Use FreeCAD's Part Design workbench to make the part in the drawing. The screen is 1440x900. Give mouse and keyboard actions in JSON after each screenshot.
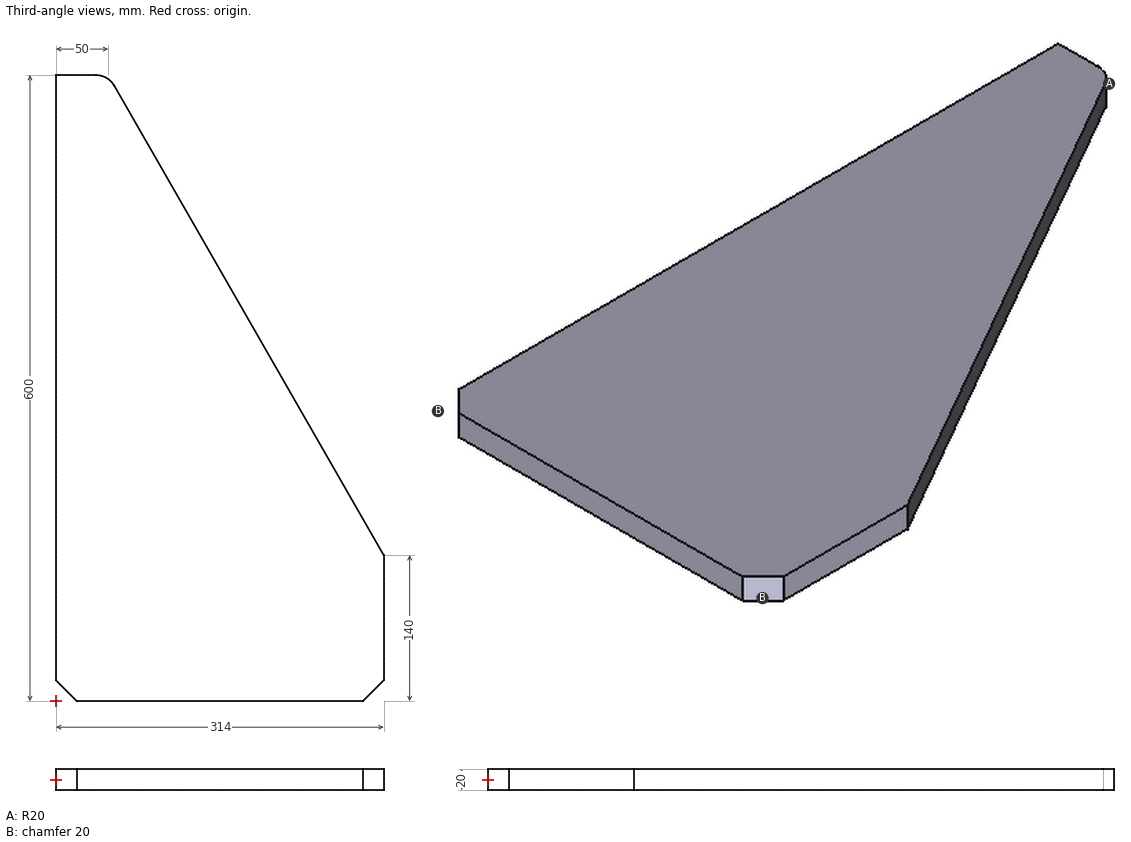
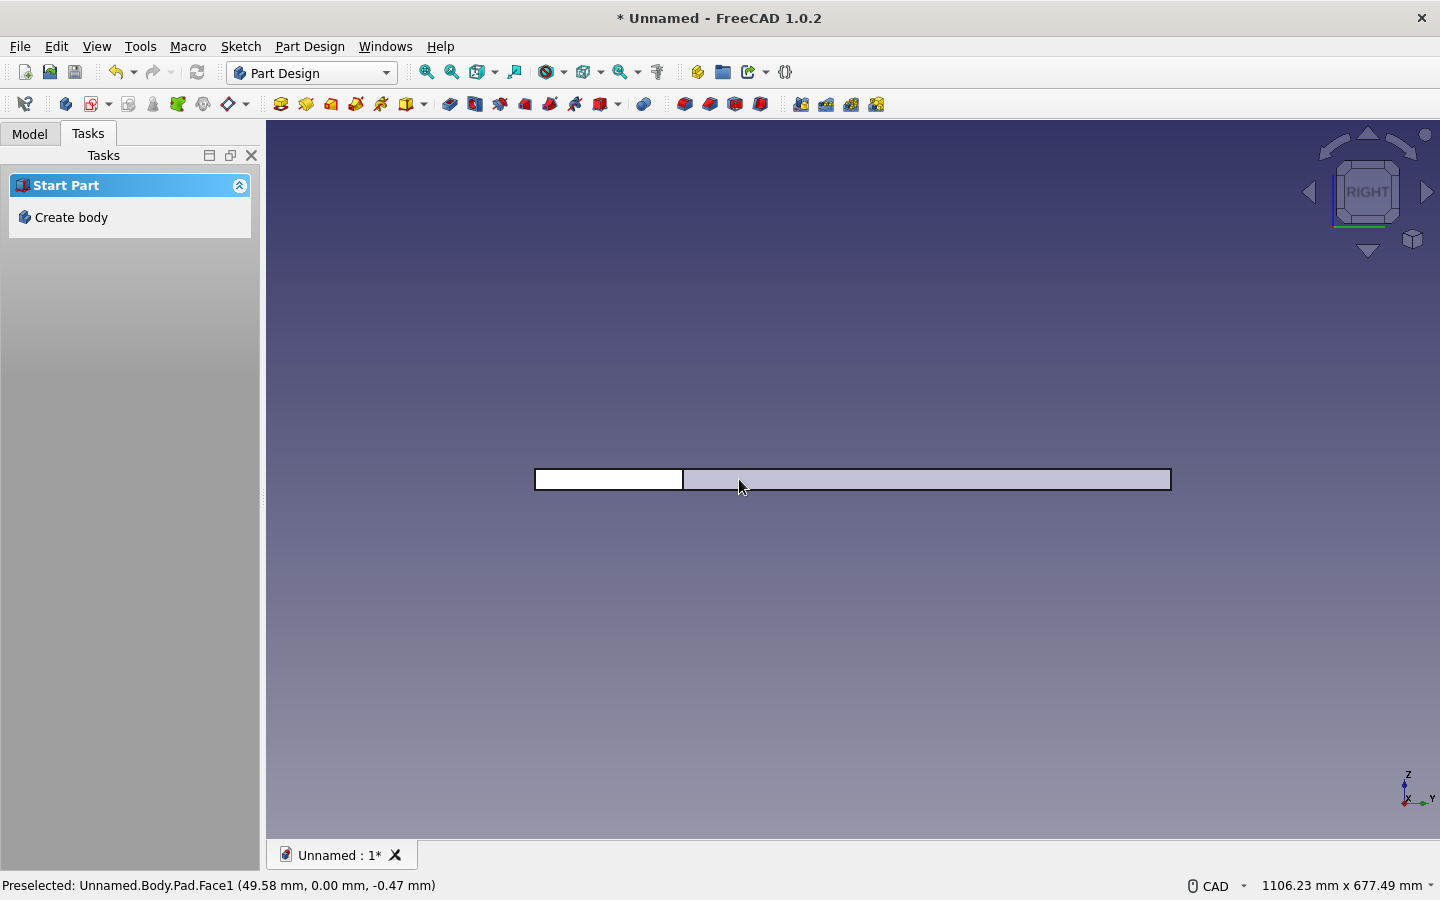
{"action": "scroll", "coordinate": [1171, 478], "scroll_direction": "up", "scroll_amount": 4}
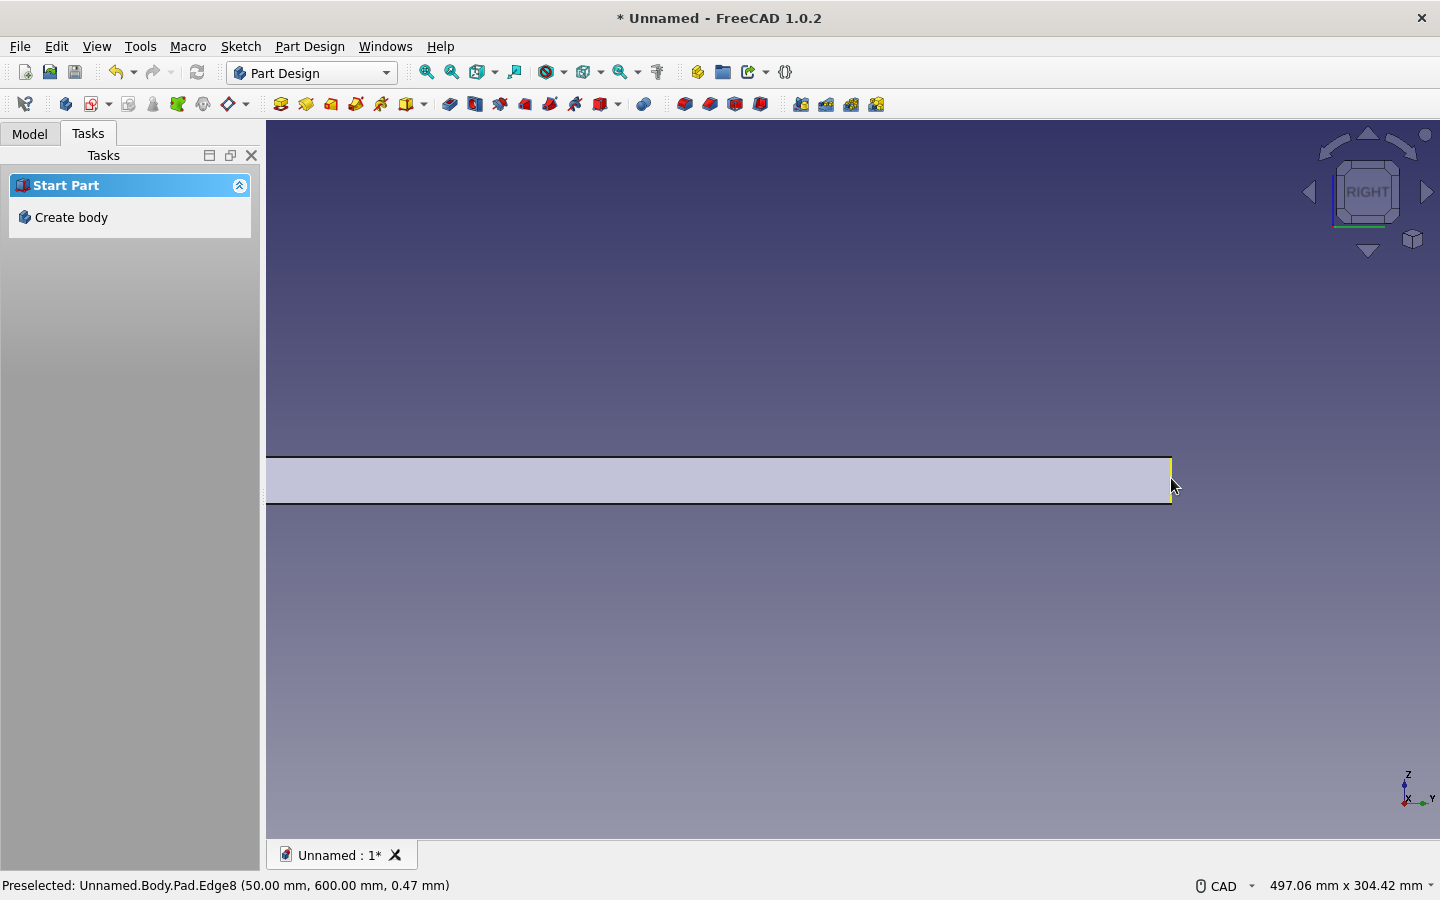
{"action": "key", "text": "v f"}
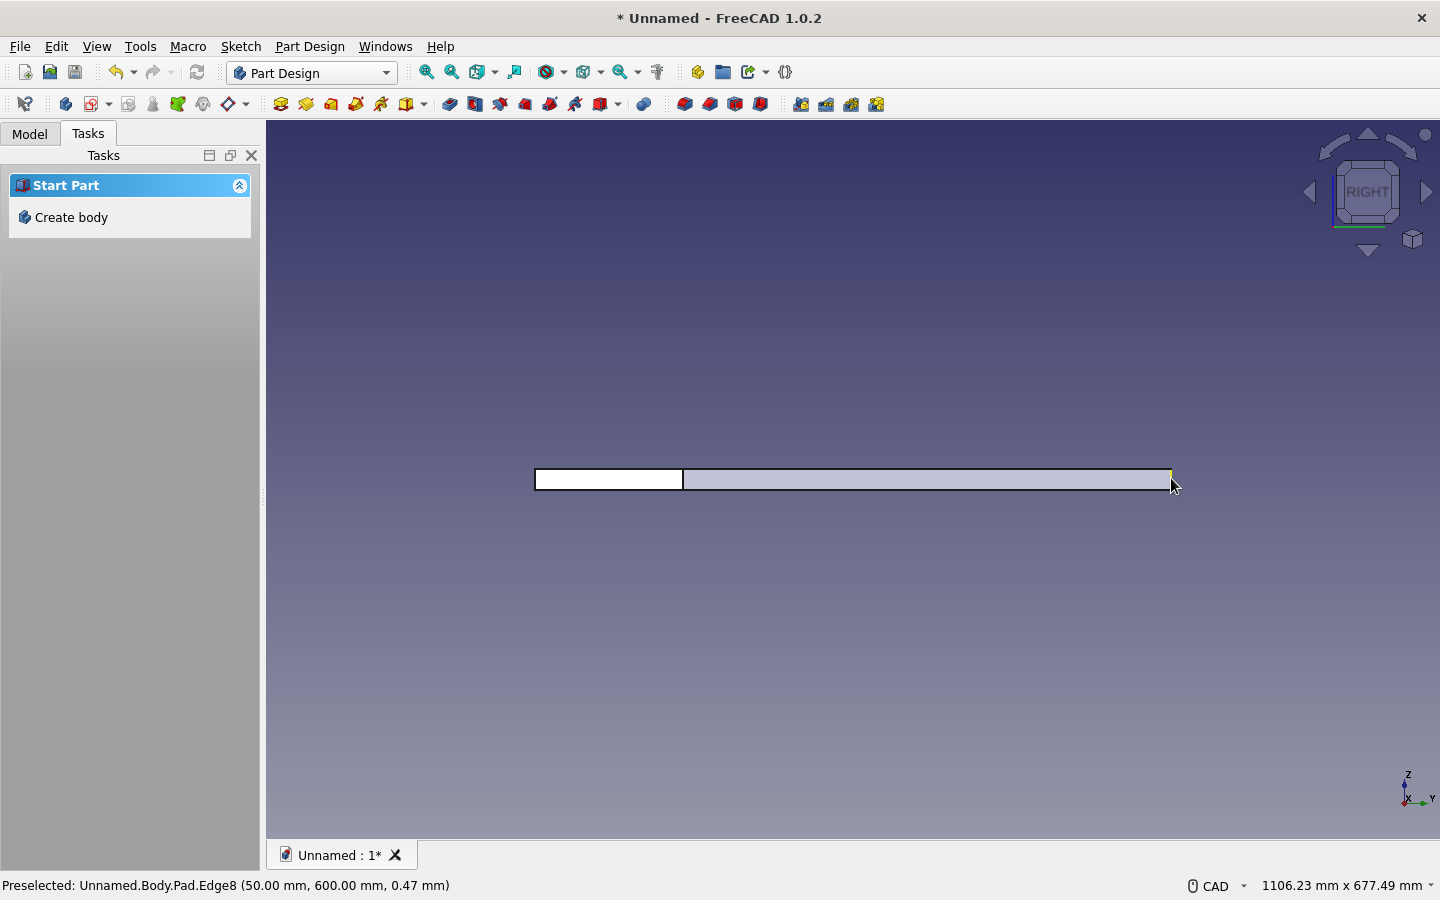
{"action": "key", "text": "5"}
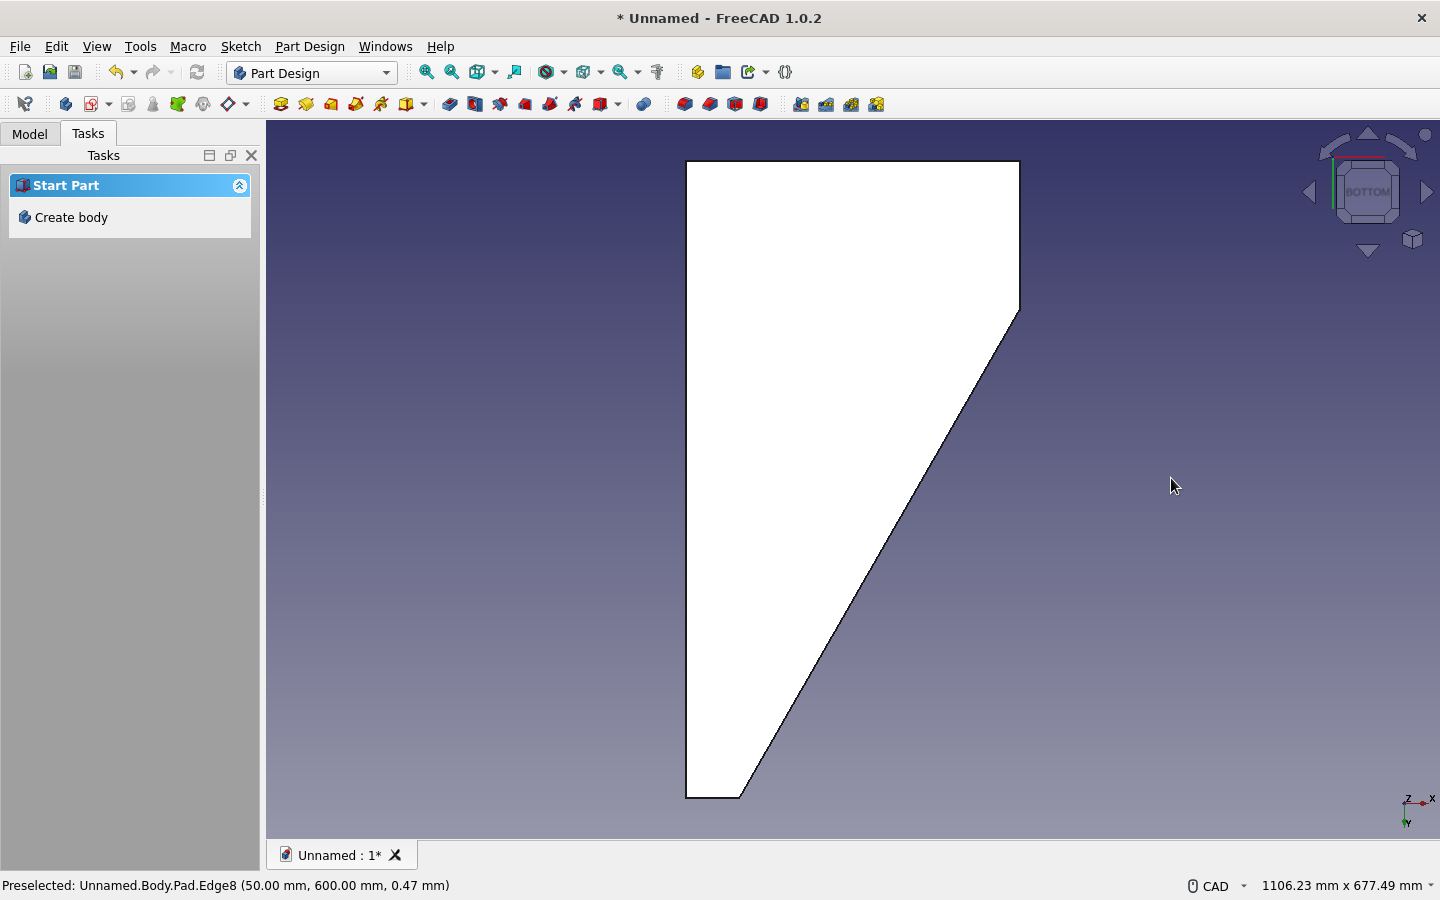
{"action": "scroll", "coordinate": [739, 797], "scroll_direction": "up", "scroll_amount": 4}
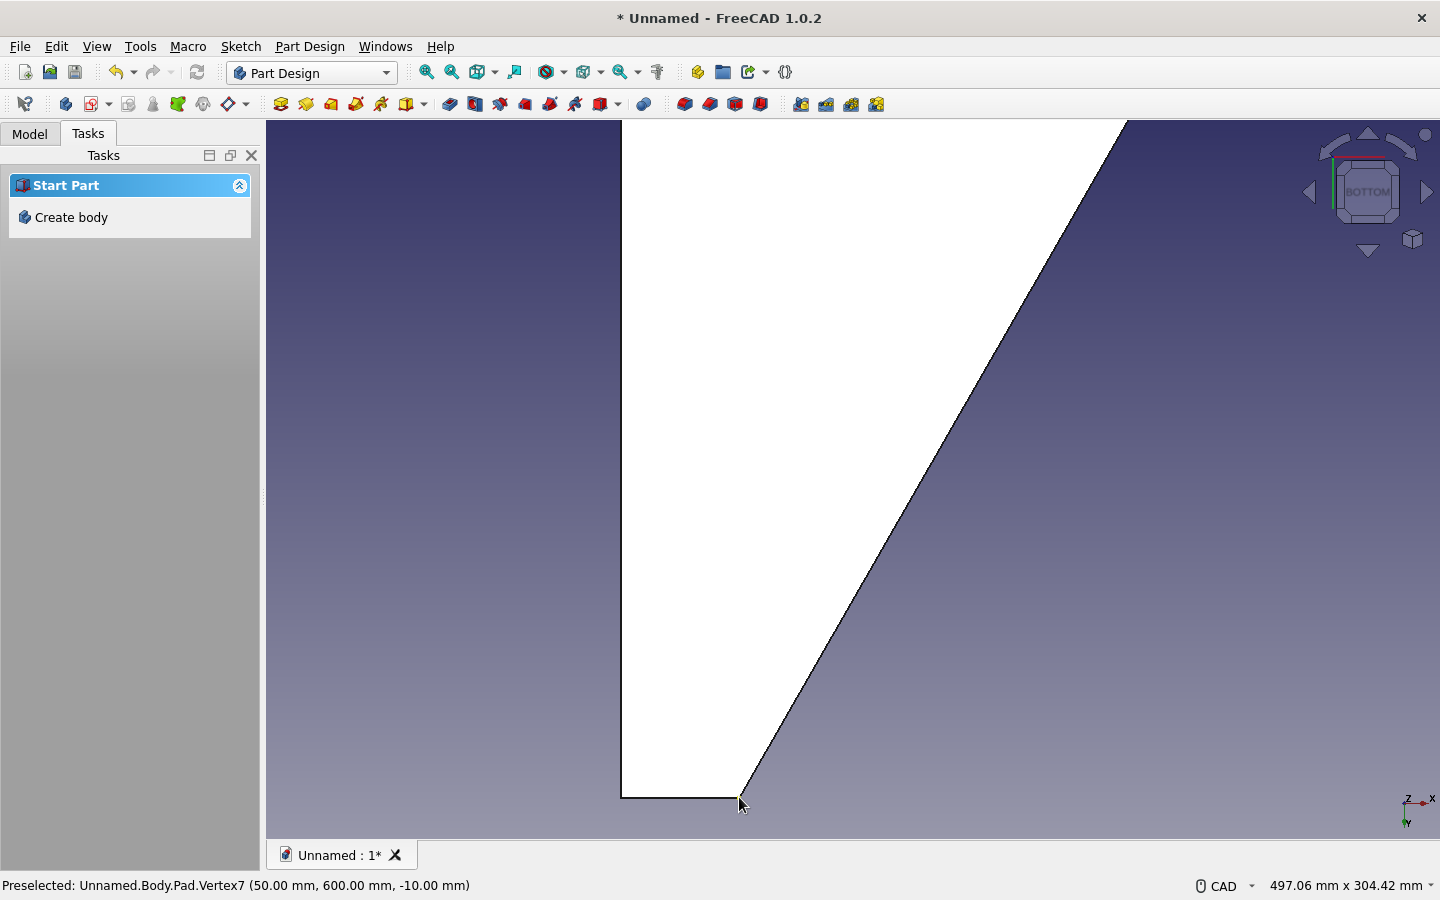
{"action": "key", "text": "v f"}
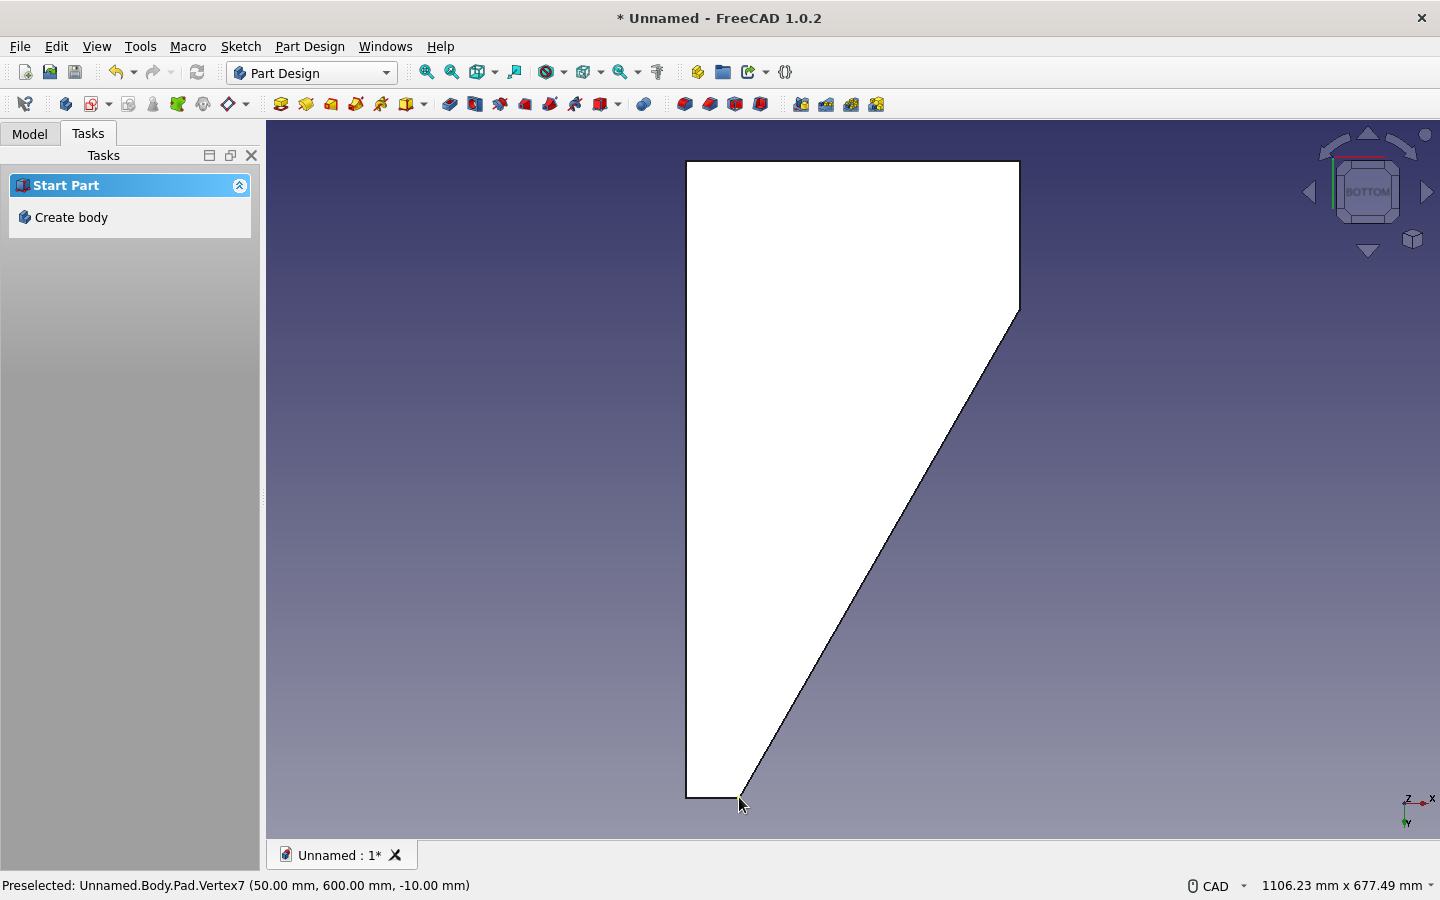
{"action": "key", "text": "4"}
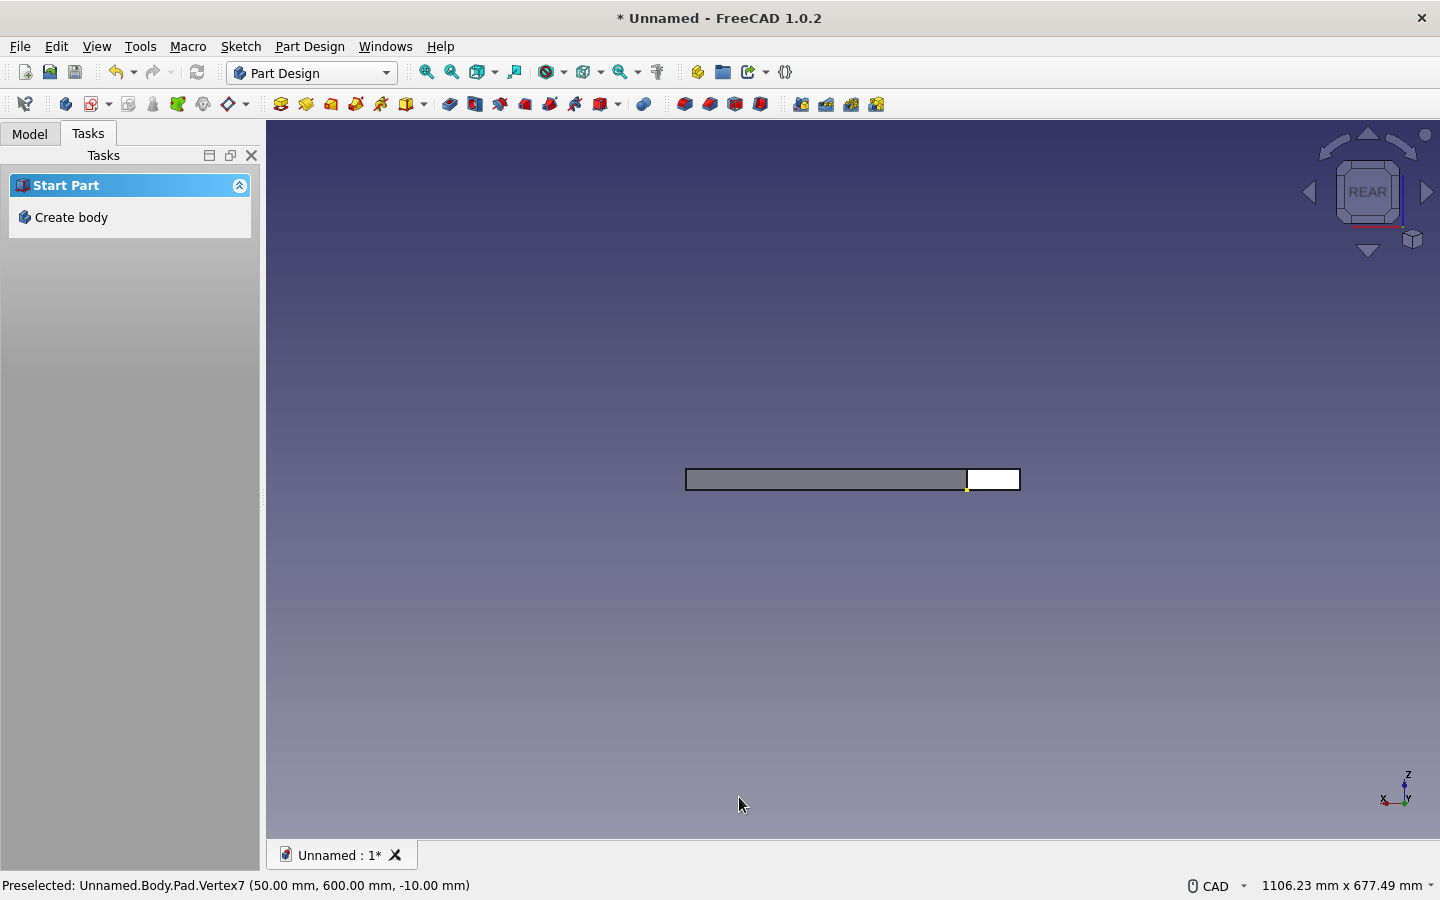
{"action": "left_click", "coordinate": [427, 72]}